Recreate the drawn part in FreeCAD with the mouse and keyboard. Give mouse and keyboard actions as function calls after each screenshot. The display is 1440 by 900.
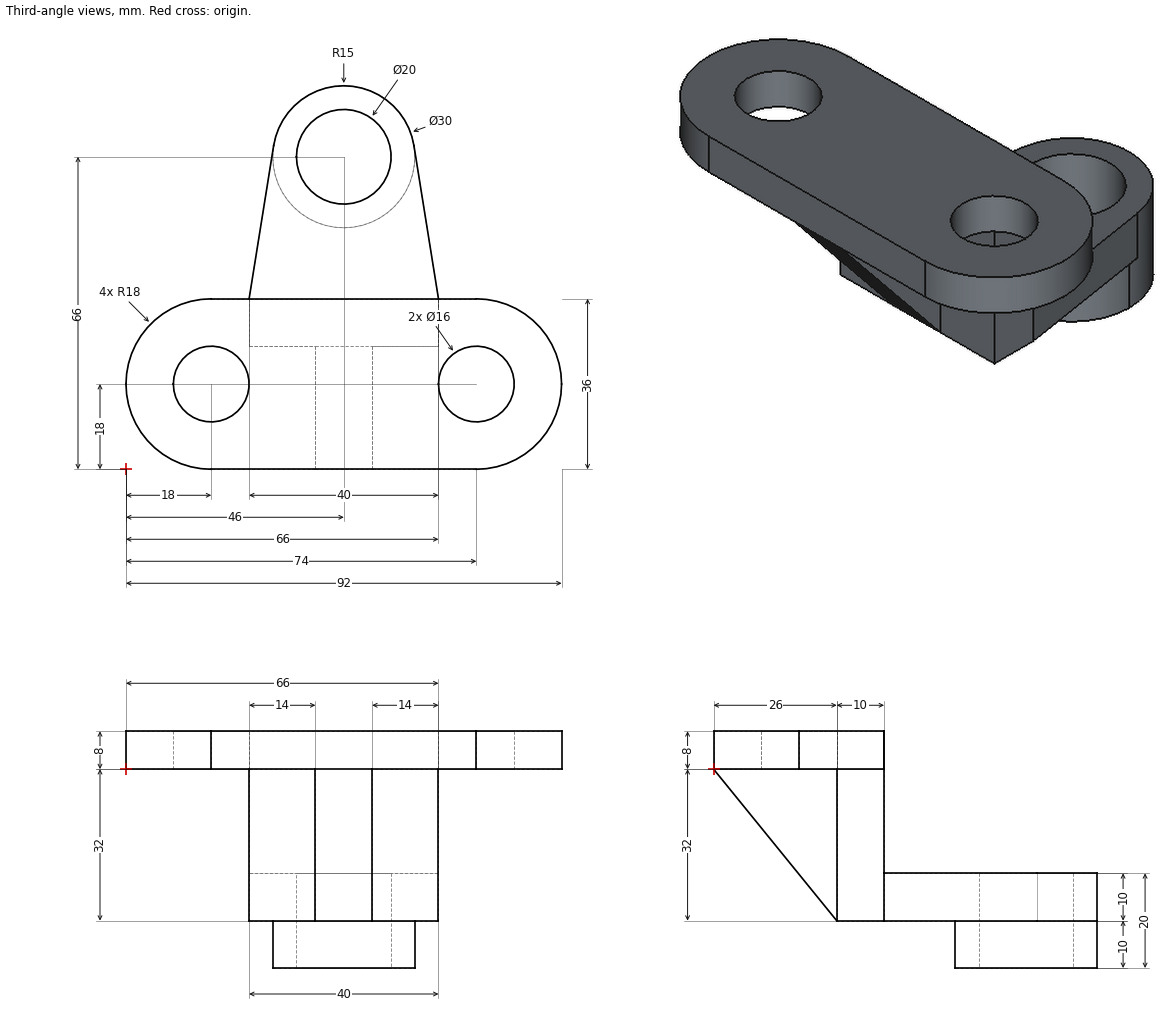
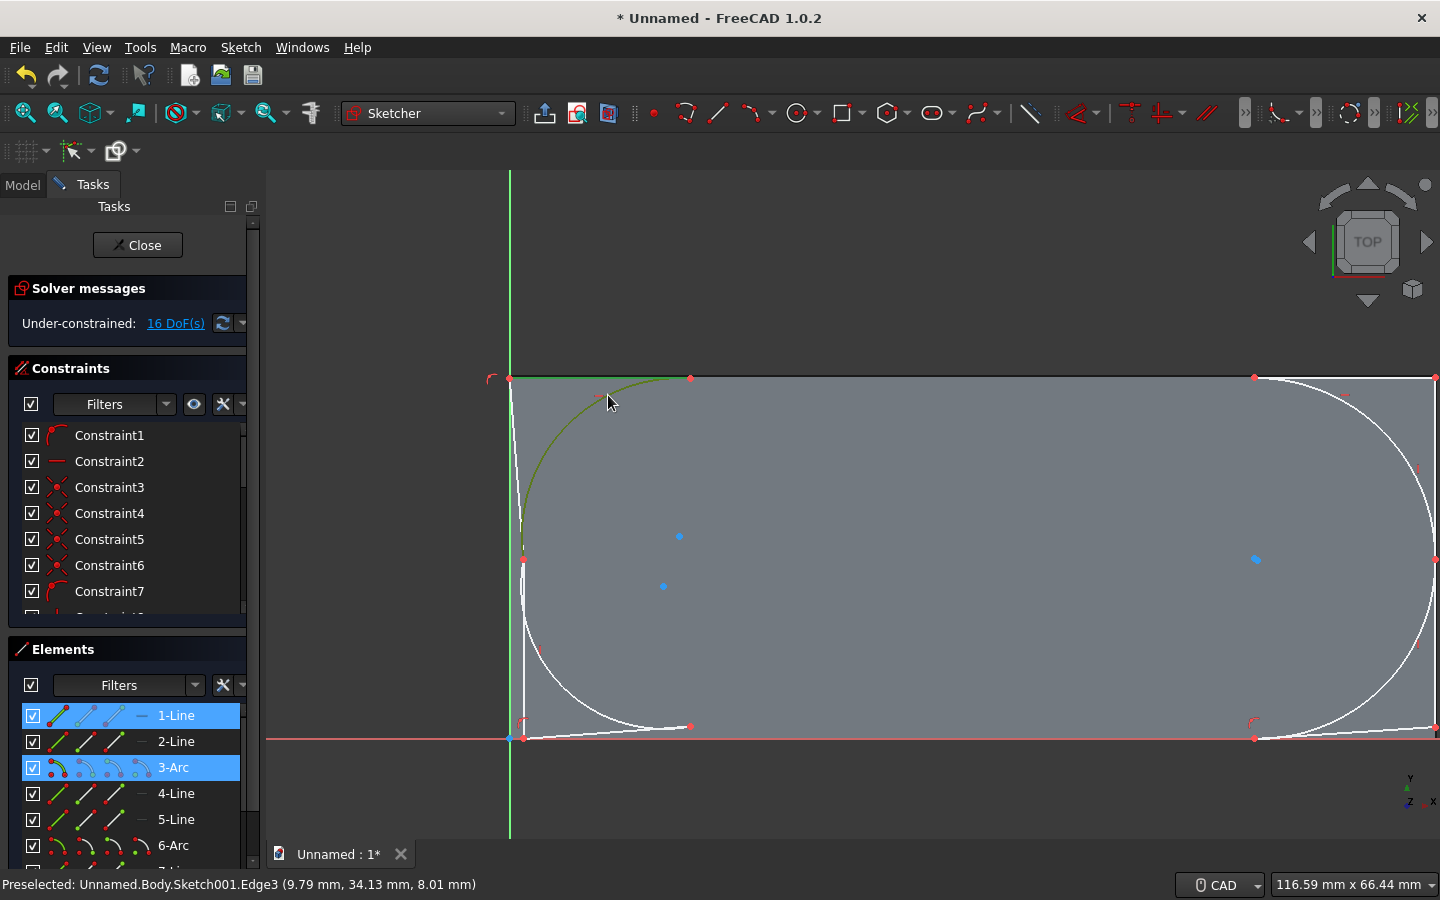
key(t)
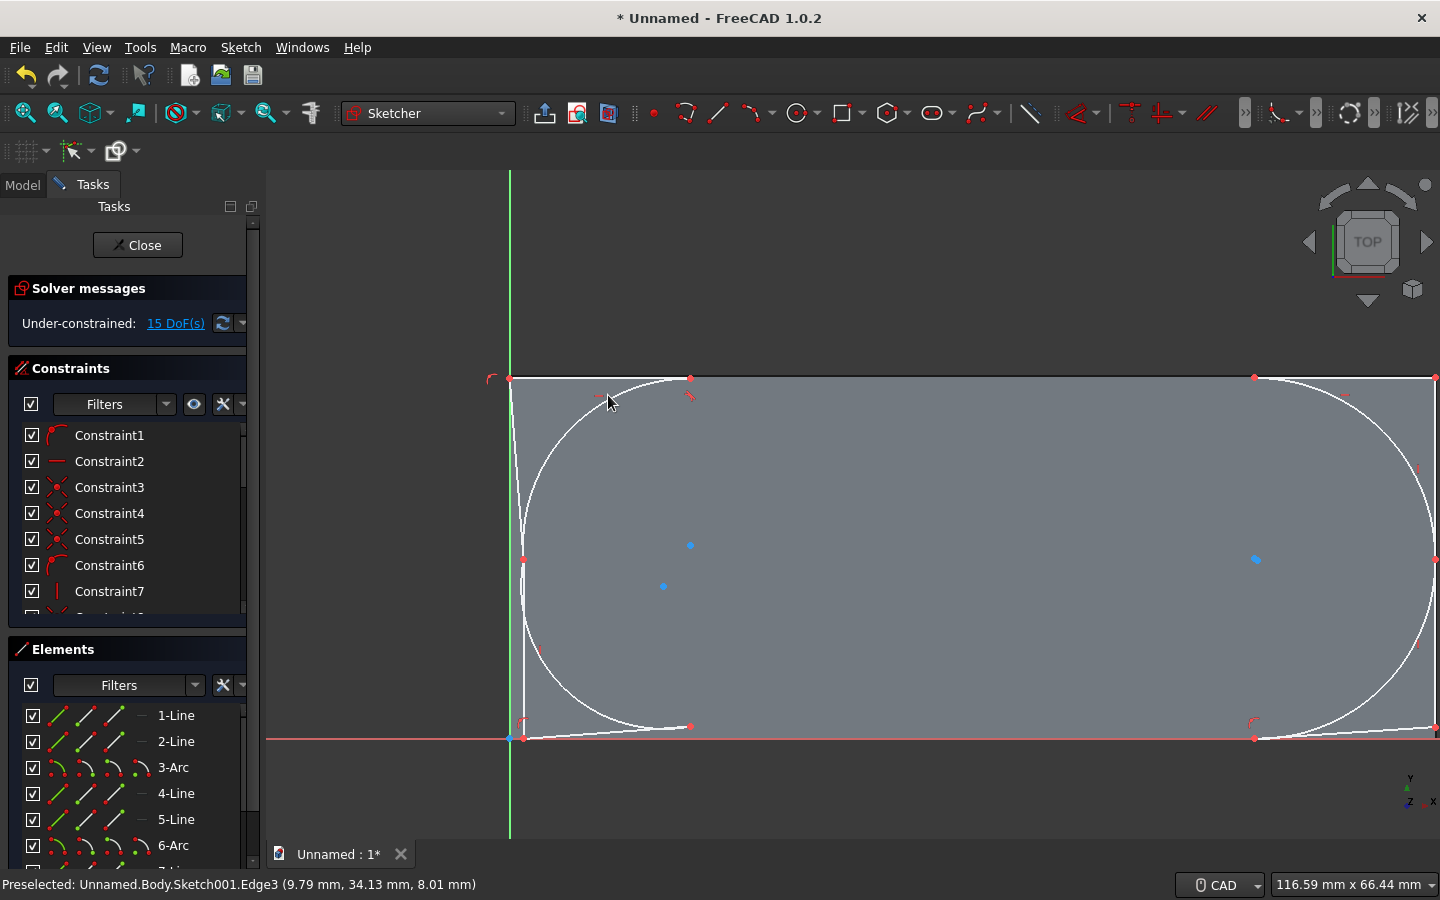
click(512, 415)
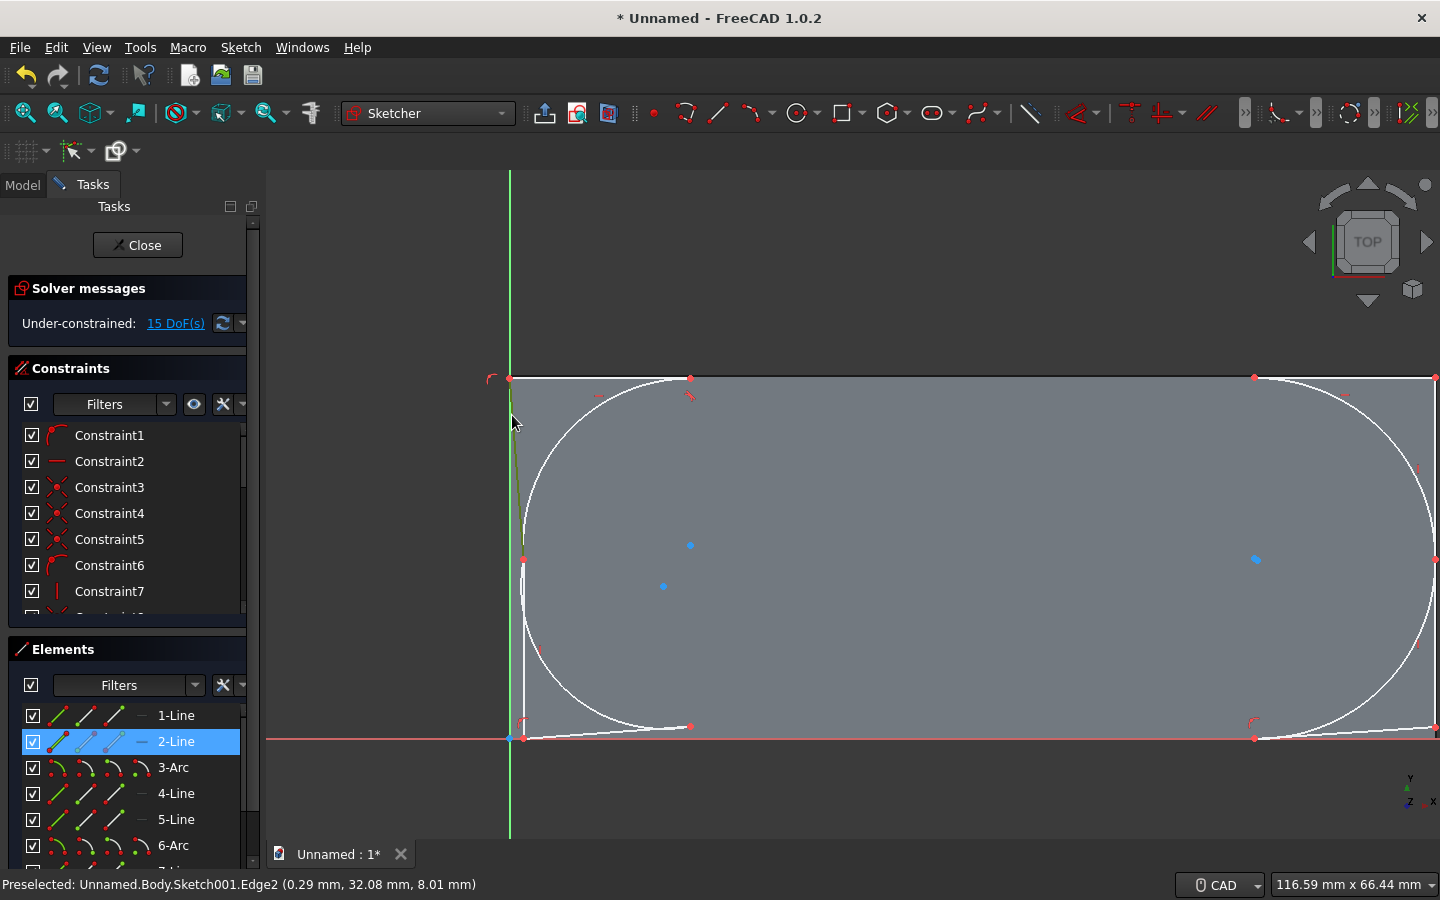
click(611, 399)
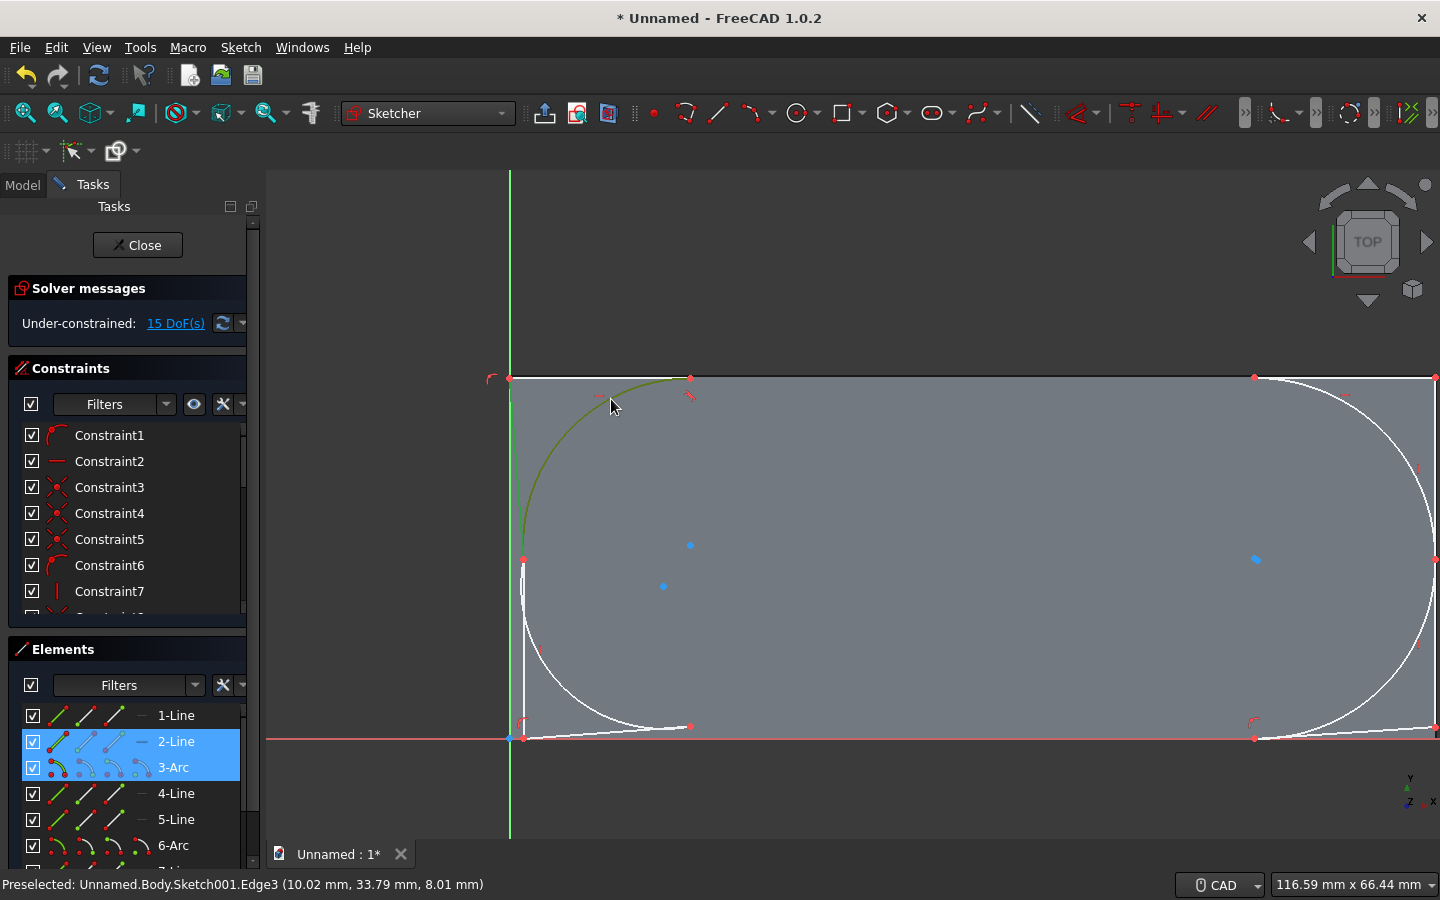
key(t)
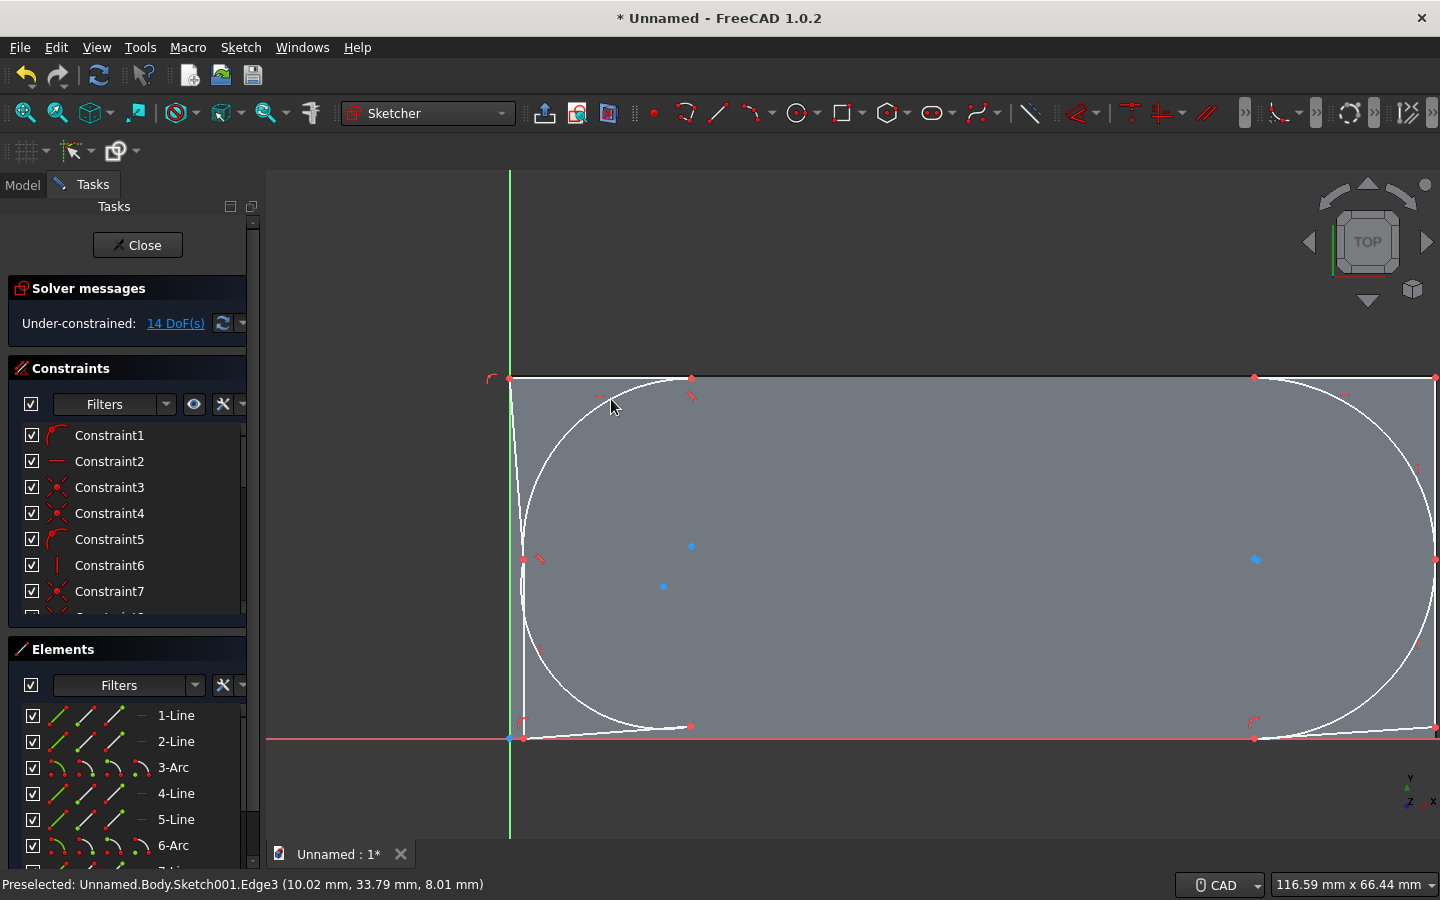
click(512, 415)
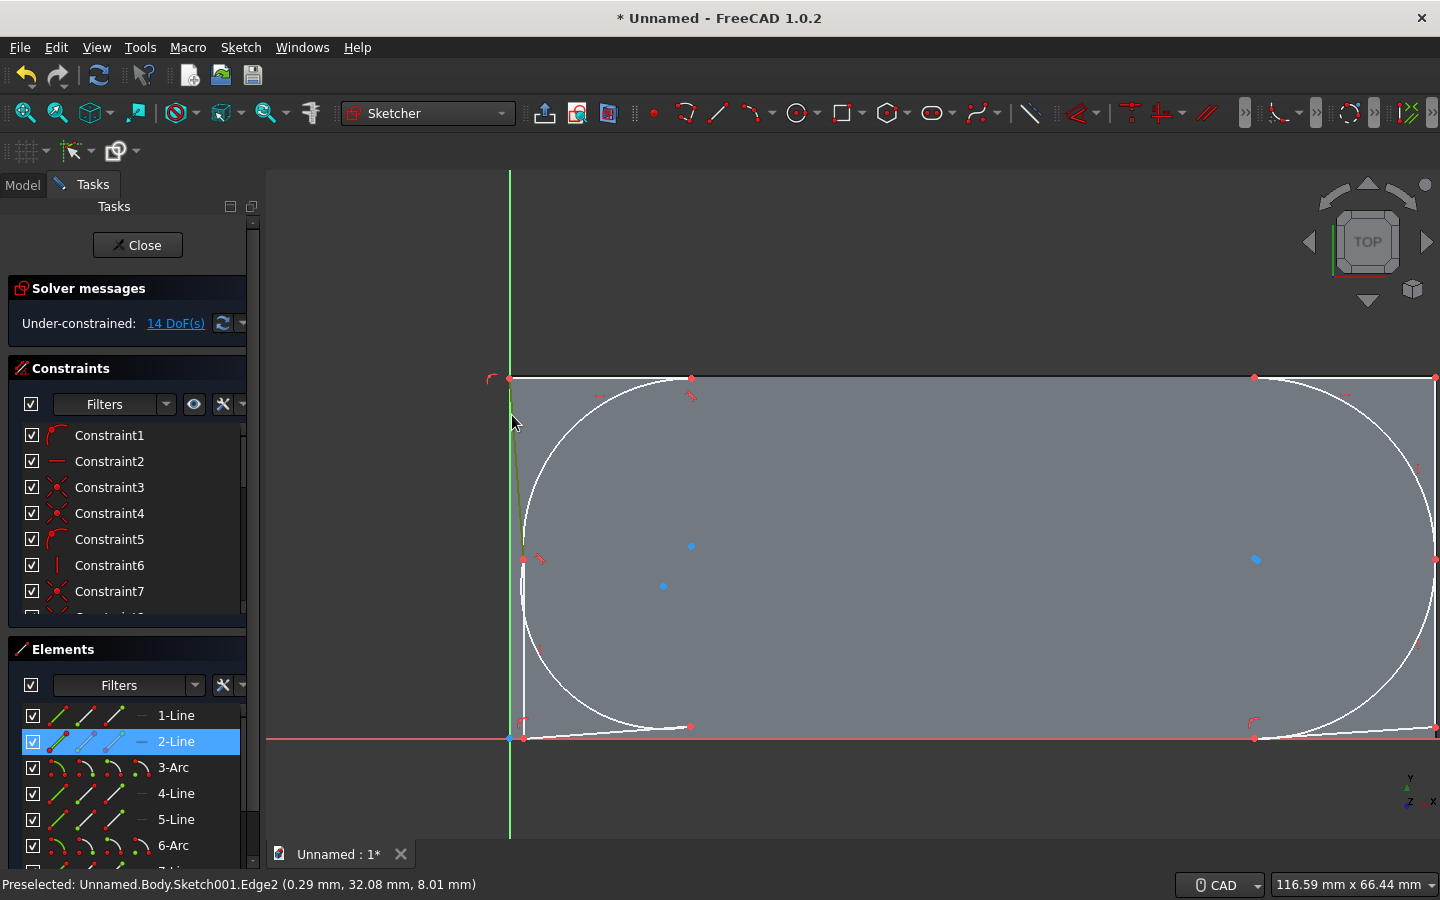
click(609, 718)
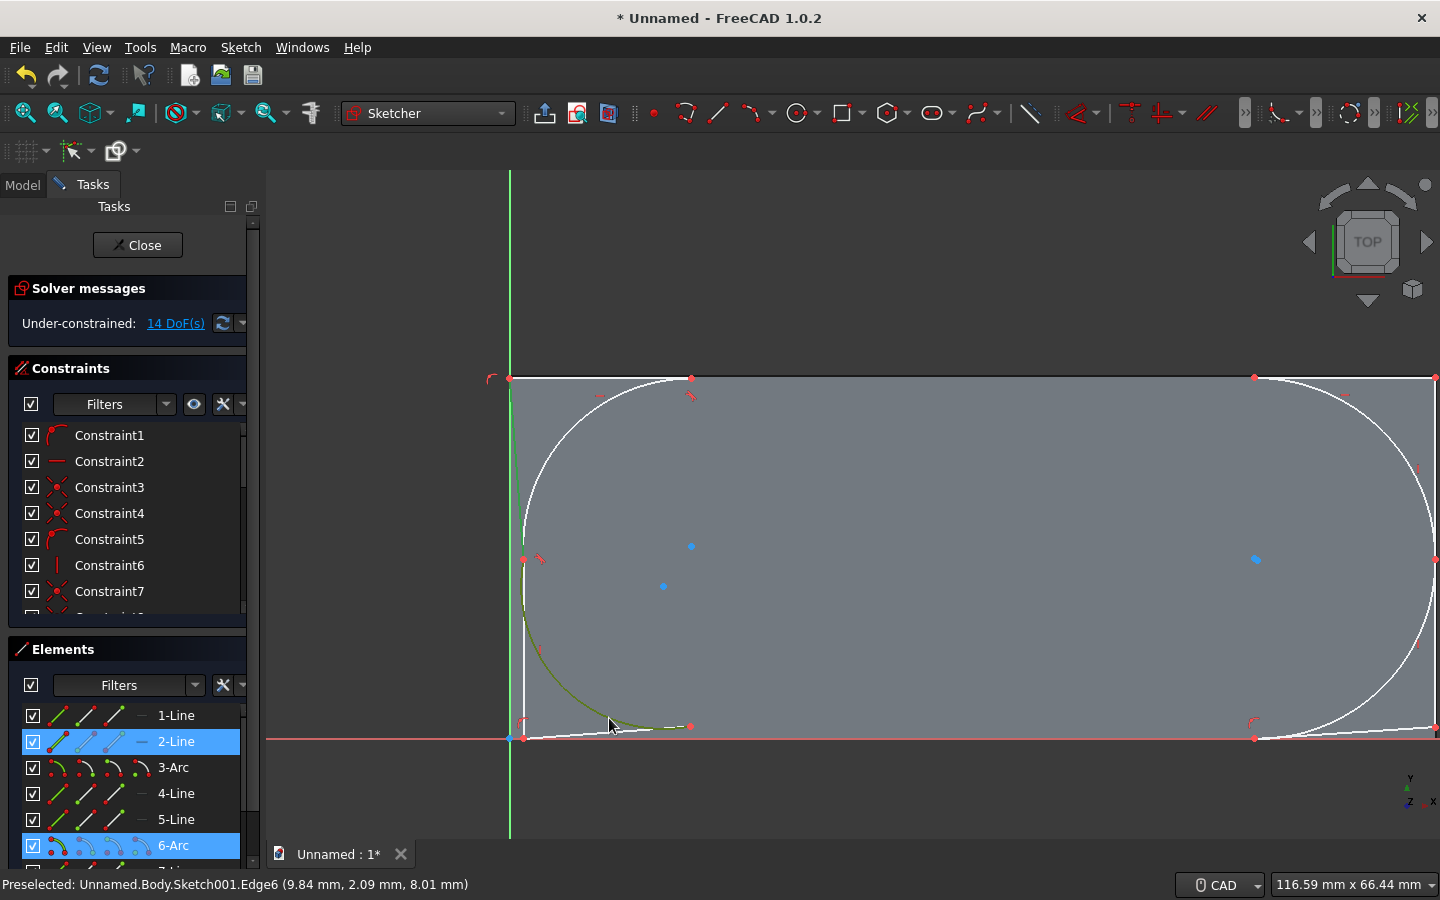
key(t)